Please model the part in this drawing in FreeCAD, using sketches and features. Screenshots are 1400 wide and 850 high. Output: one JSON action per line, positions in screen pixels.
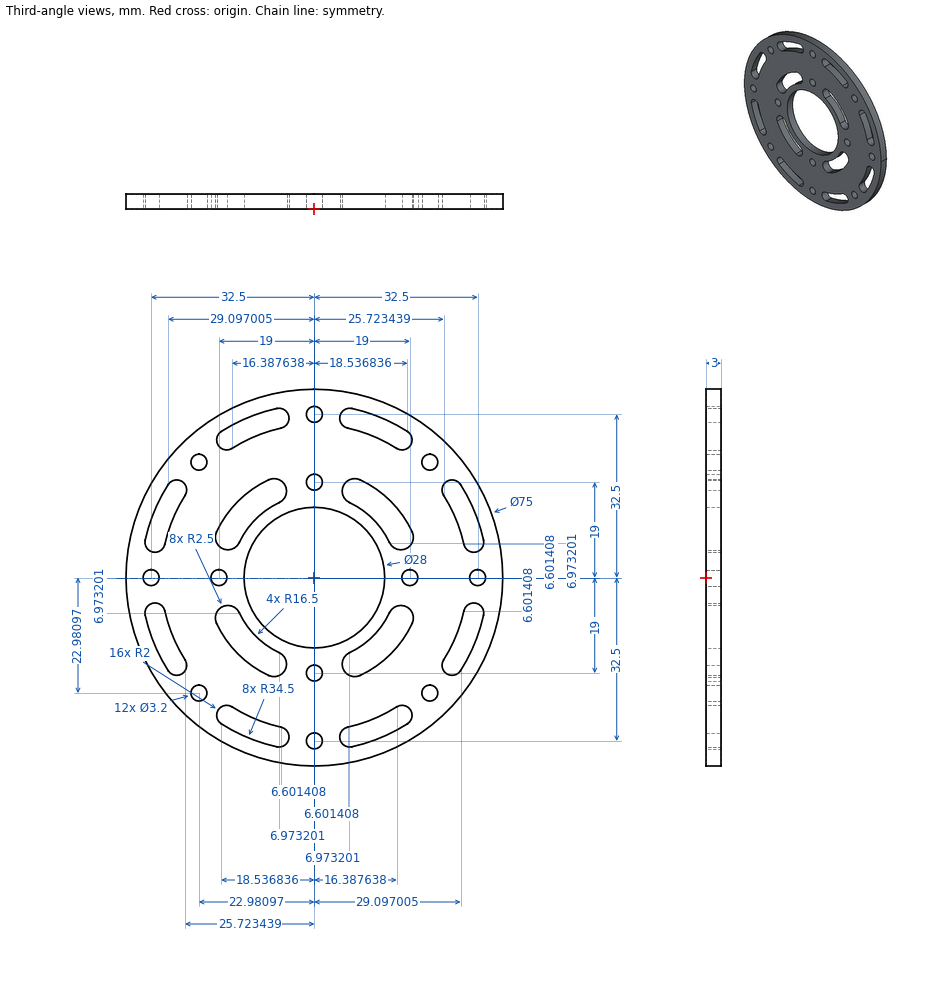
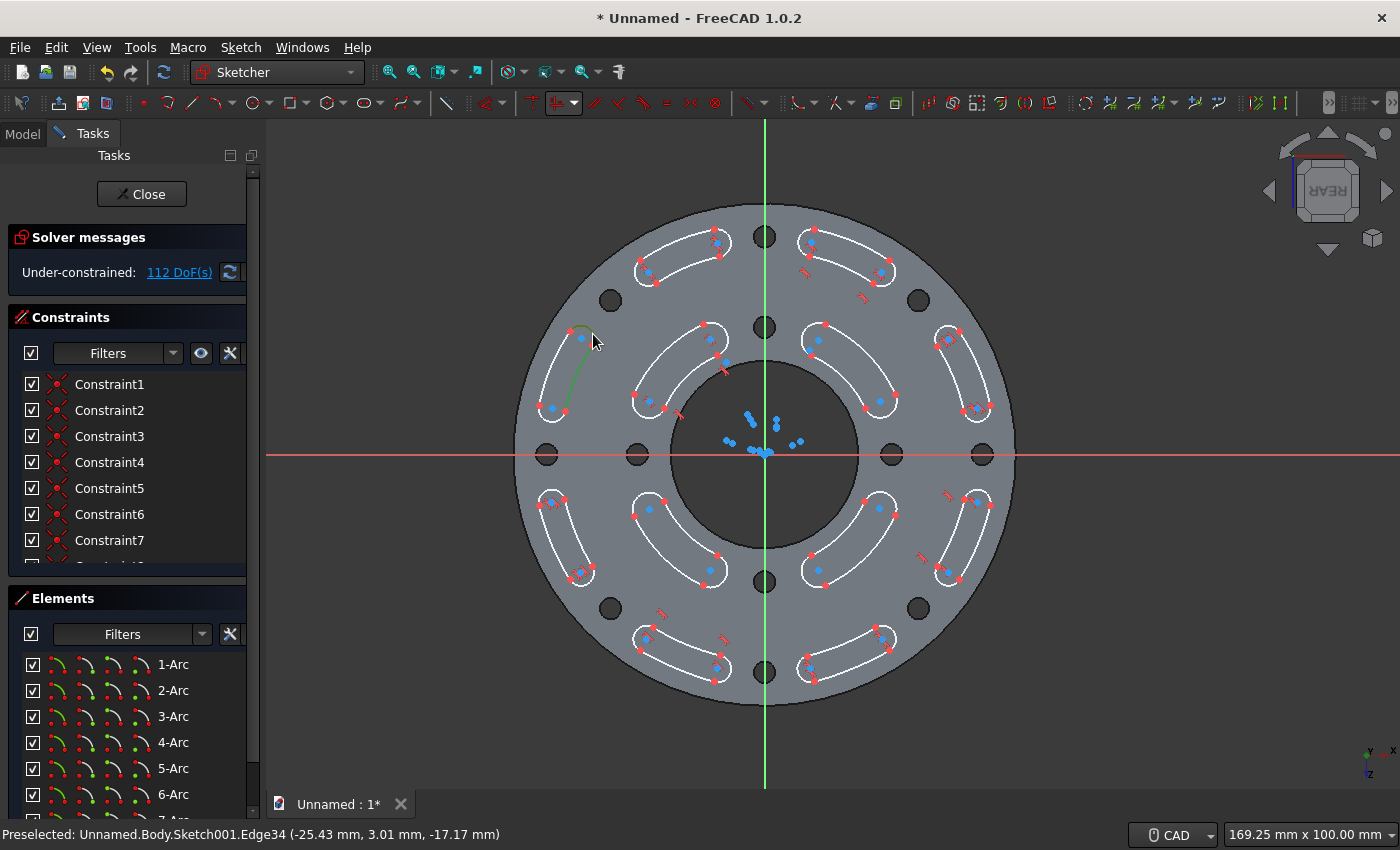
{"action": "left_click", "coordinate": [644, 104]}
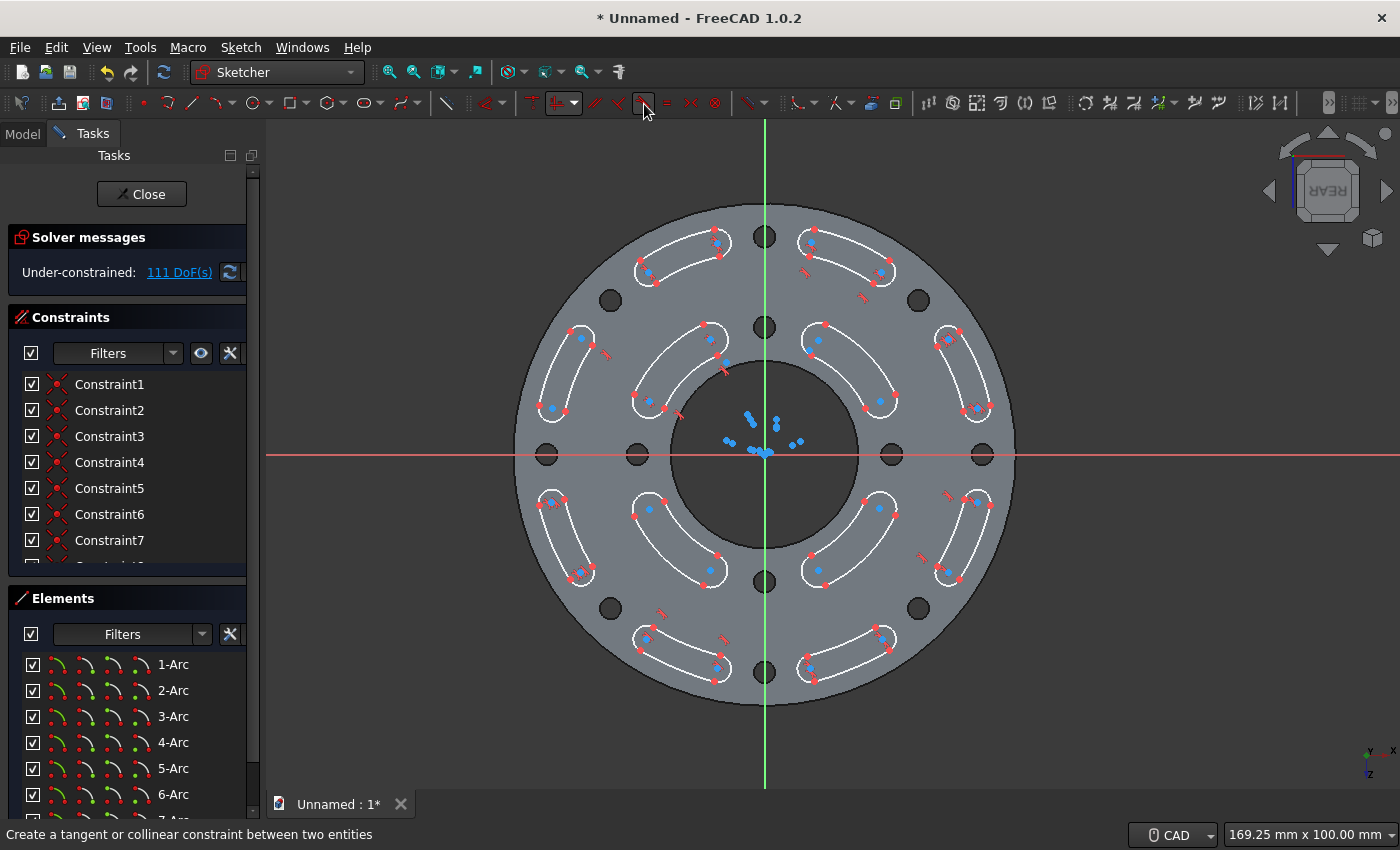
{"action": "left_click", "coordinate": [581, 364]}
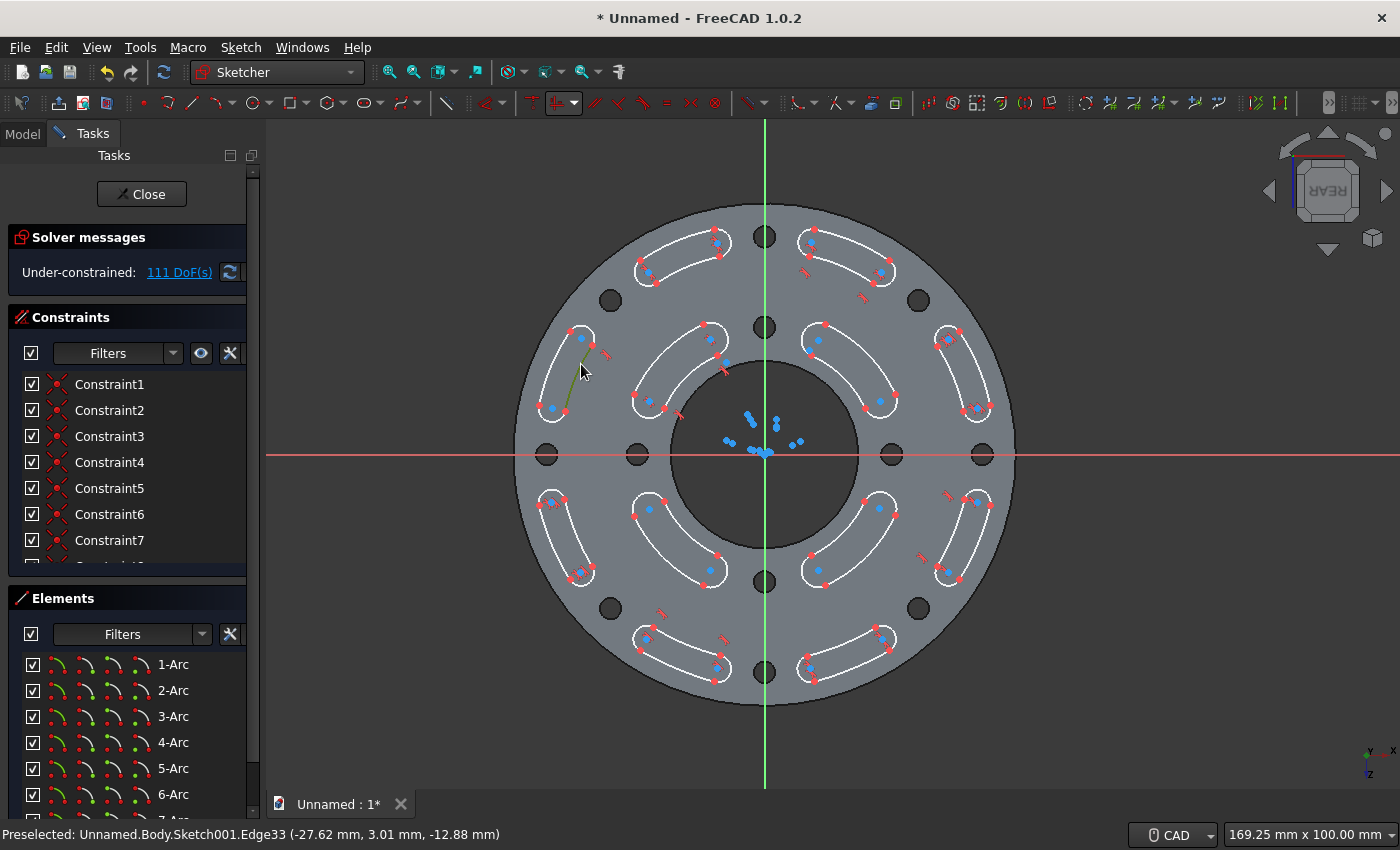
{"action": "left_click", "coordinate": [542, 417]}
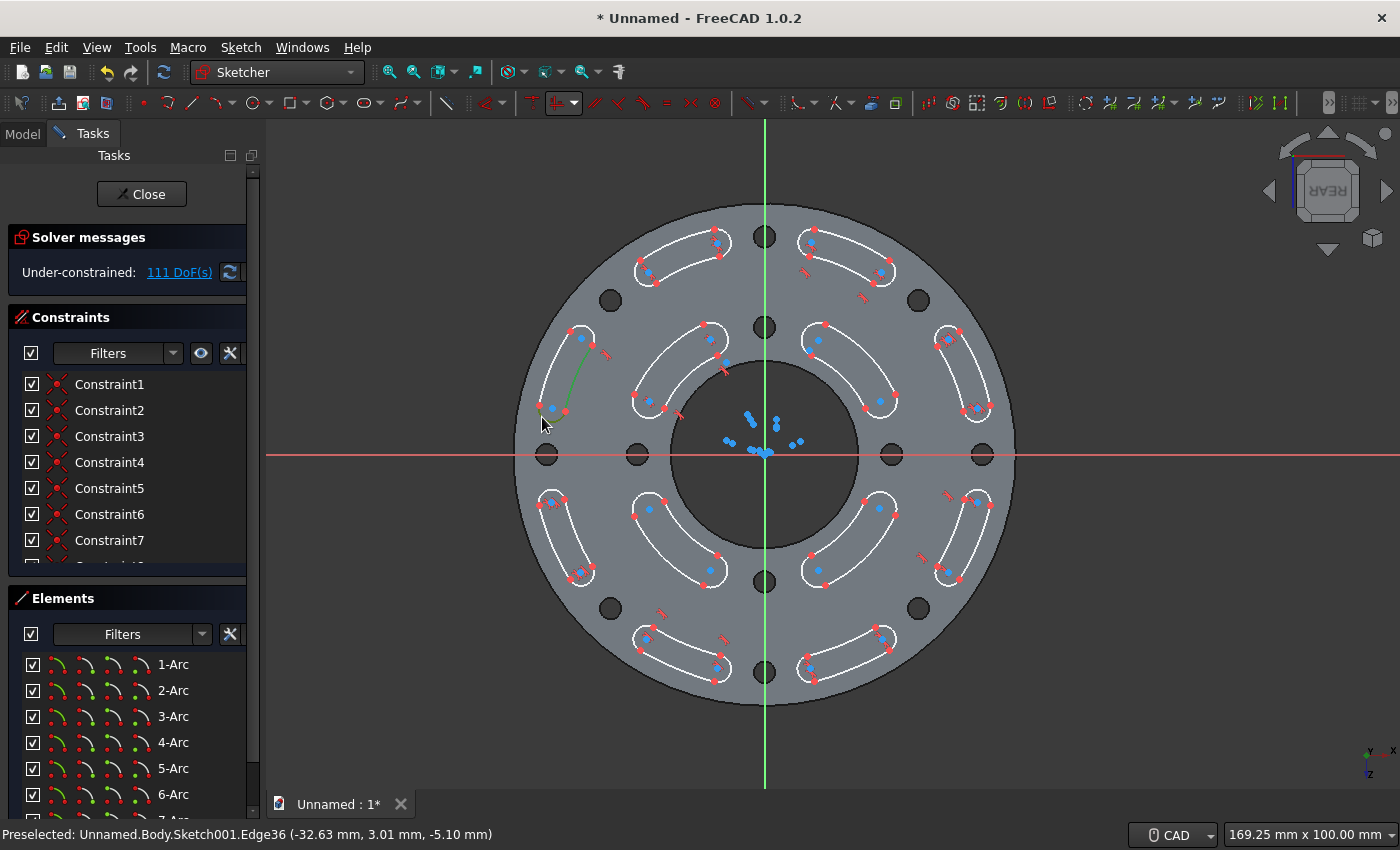
{"action": "left_click", "coordinate": [644, 104]}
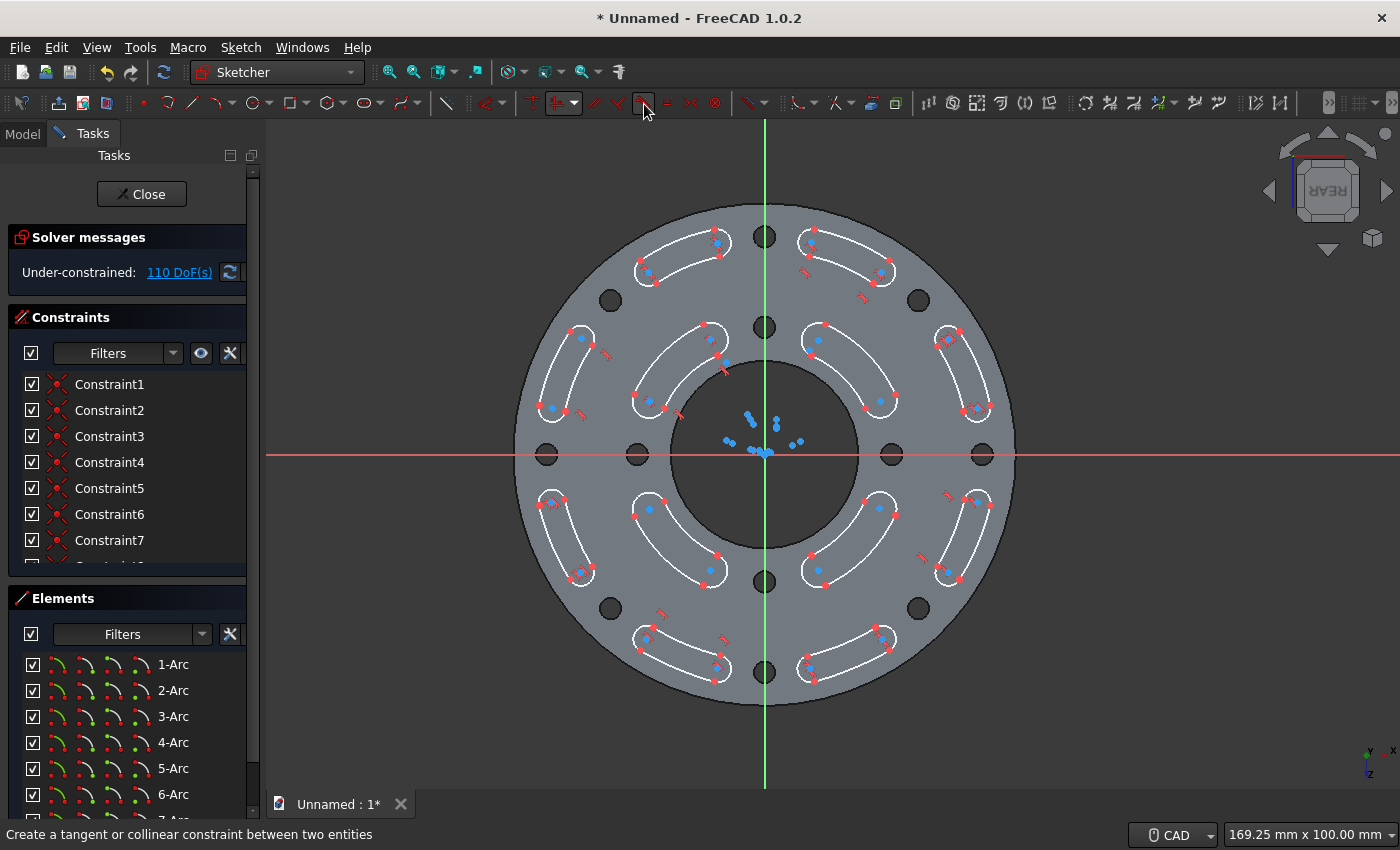
{"action": "left_click", "coordinate": [593, 334]}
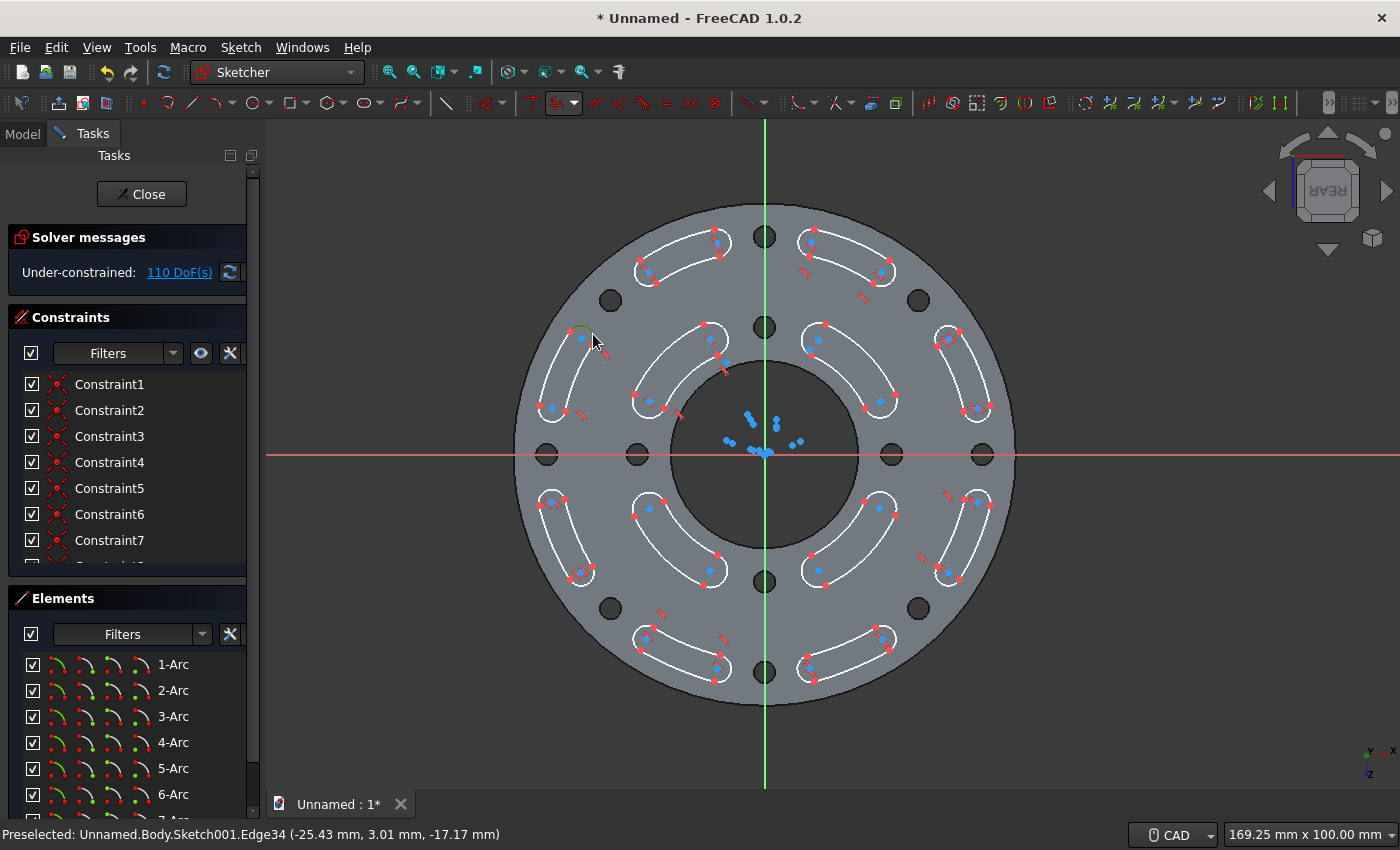
{"action": "left_click", "coordinate": [558, 352]}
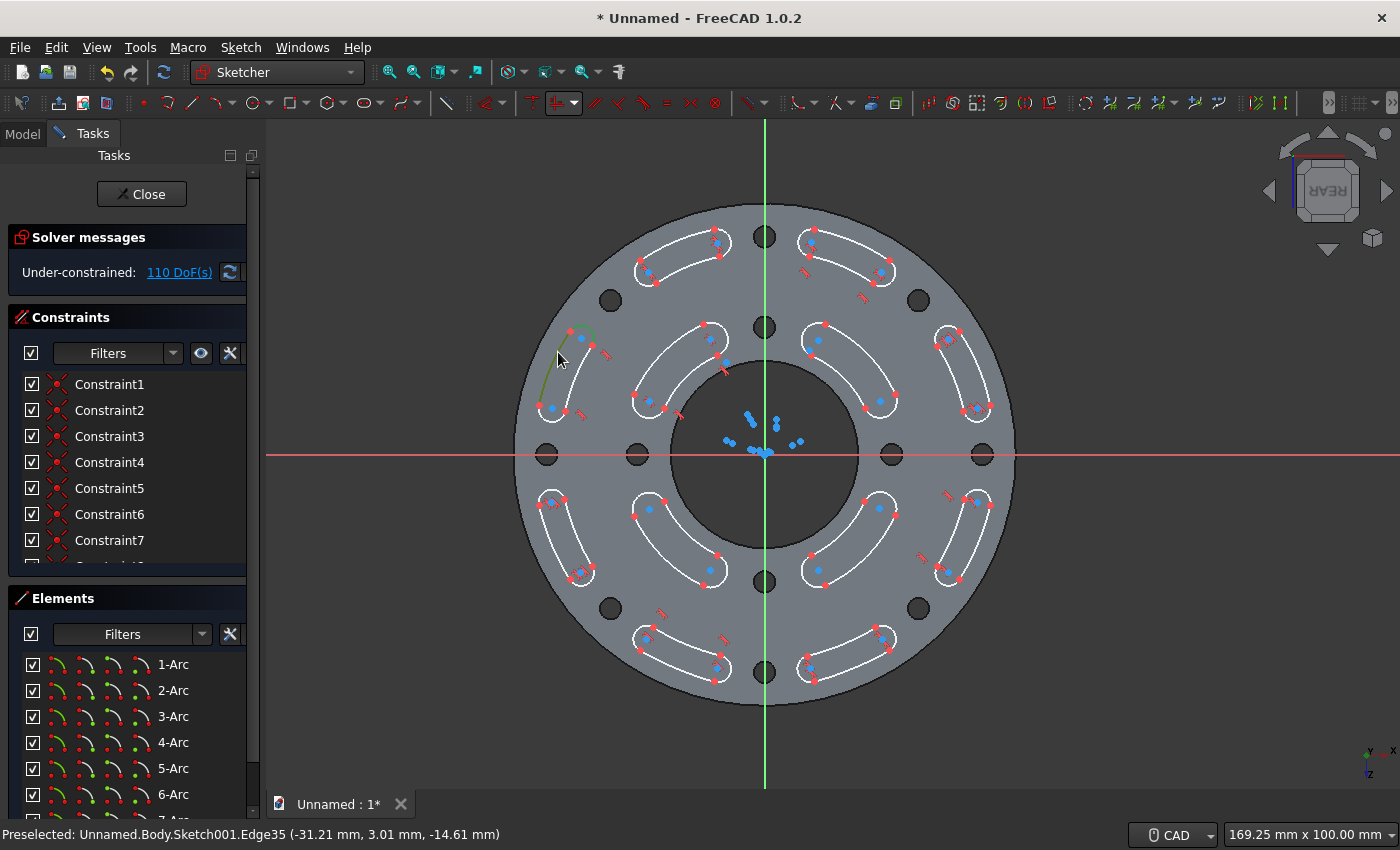
{"action": "left_click", "coordinate": [644, 104]}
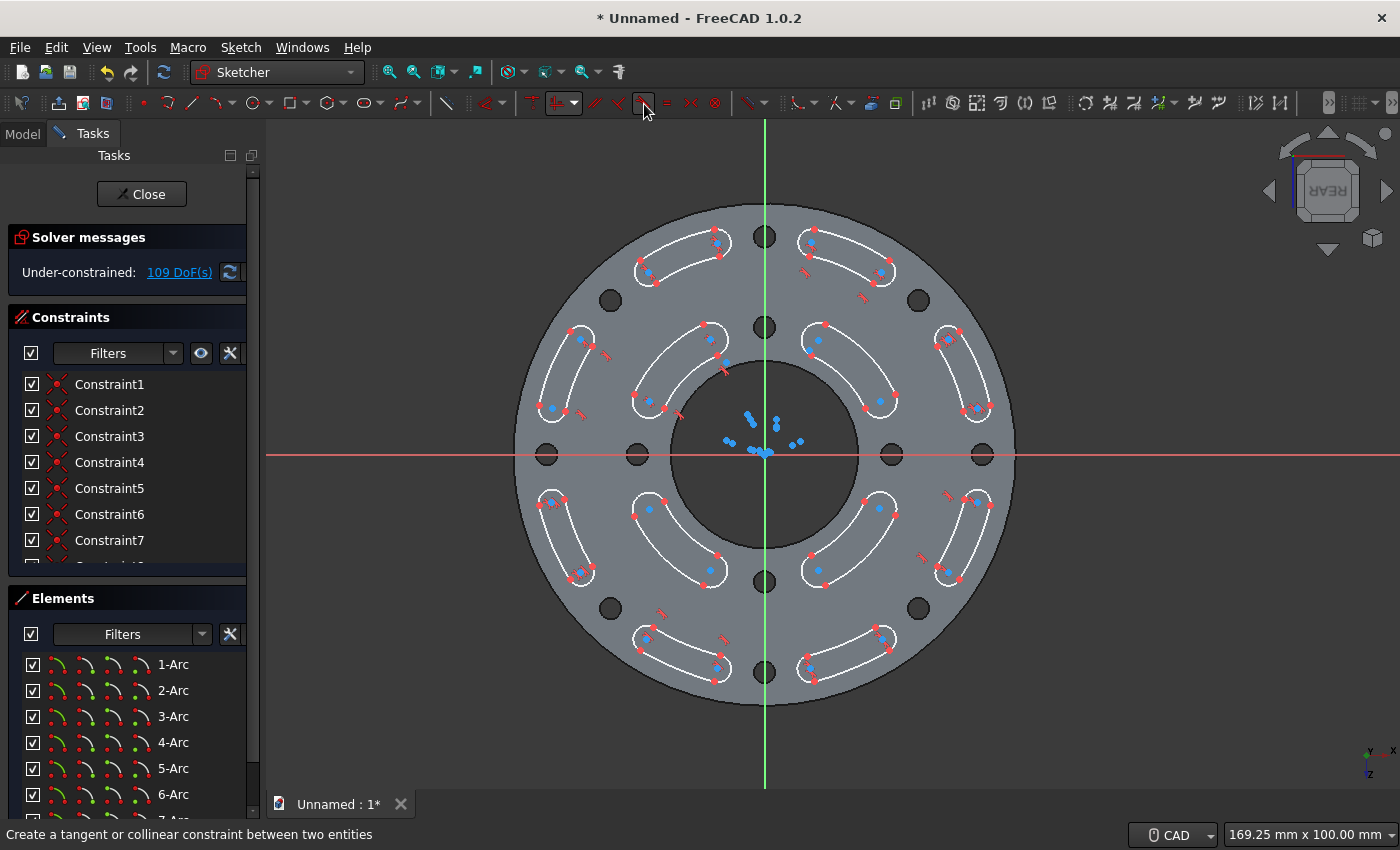
{"action": "left_click", "coordinate": [558, 352]}